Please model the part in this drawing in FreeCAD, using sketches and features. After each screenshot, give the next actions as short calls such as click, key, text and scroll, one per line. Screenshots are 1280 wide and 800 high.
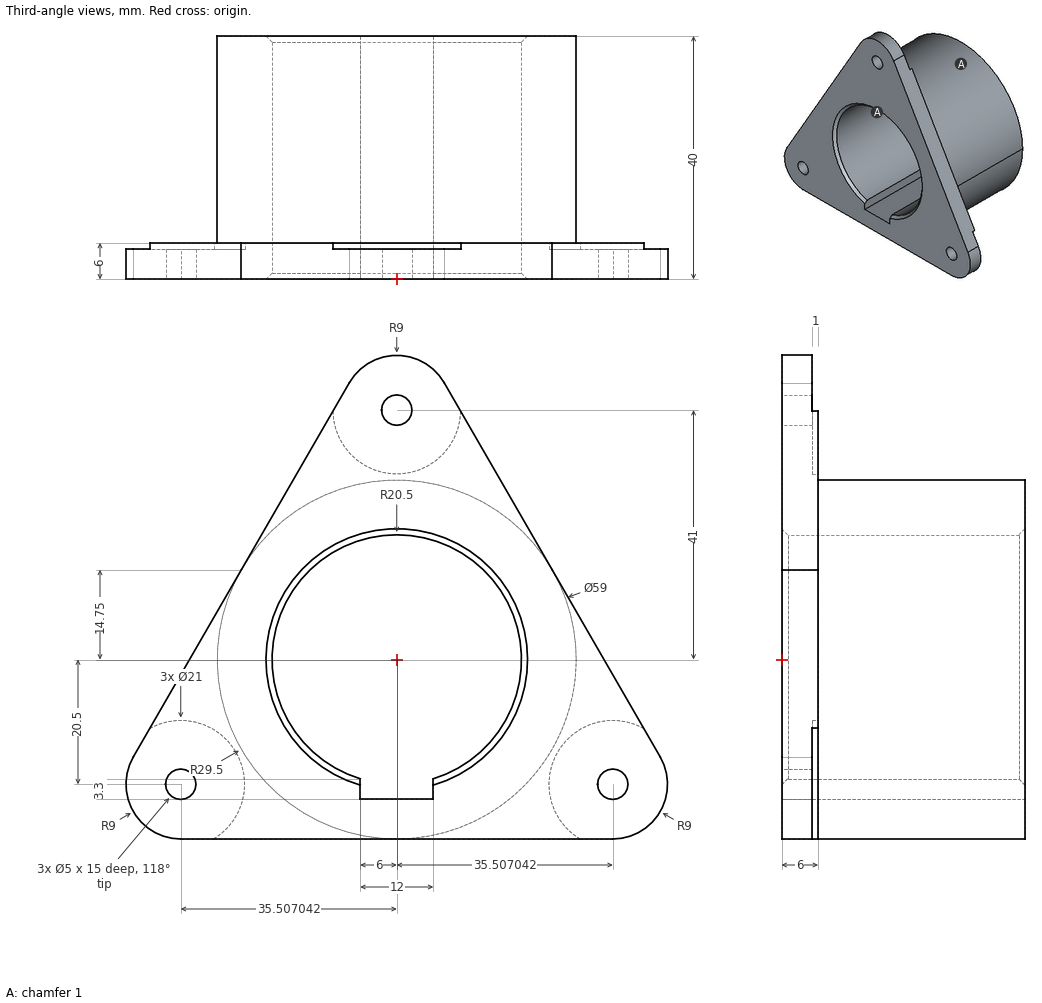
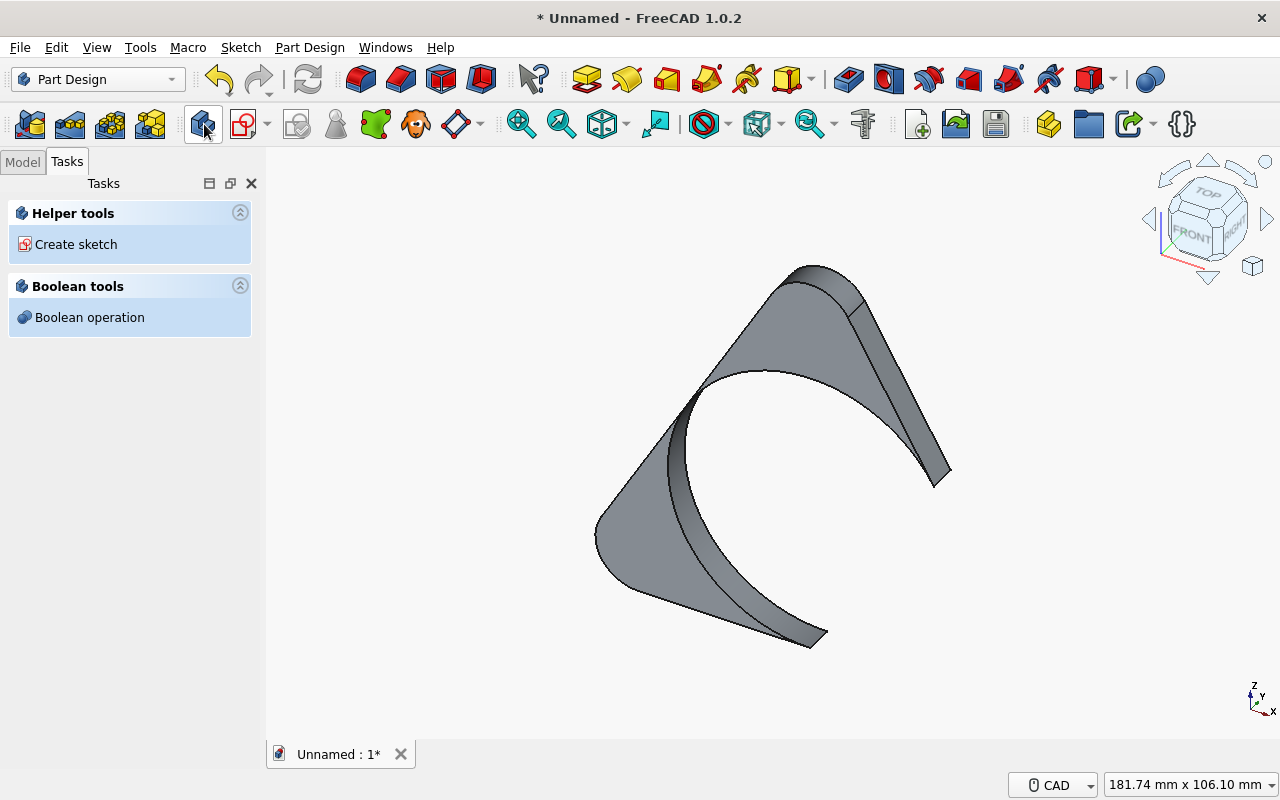
click(306, 699)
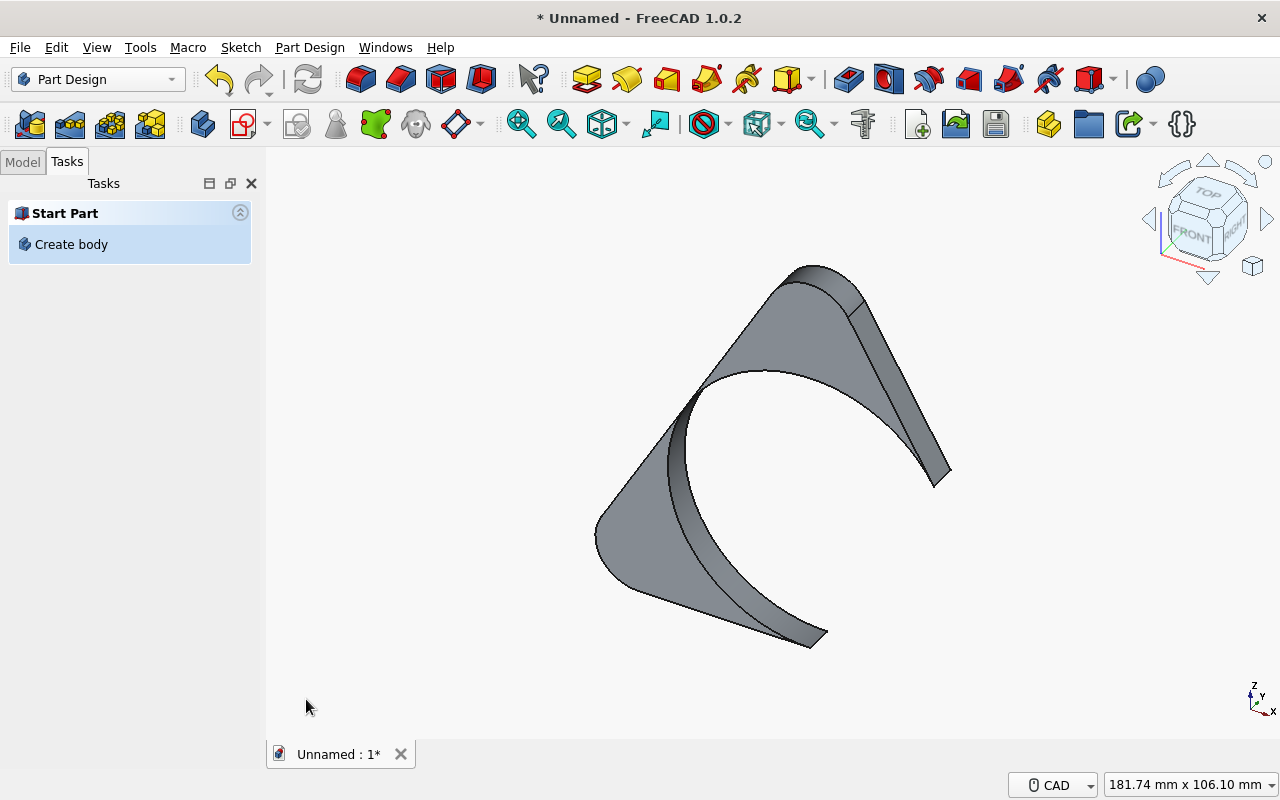
click(244, 124)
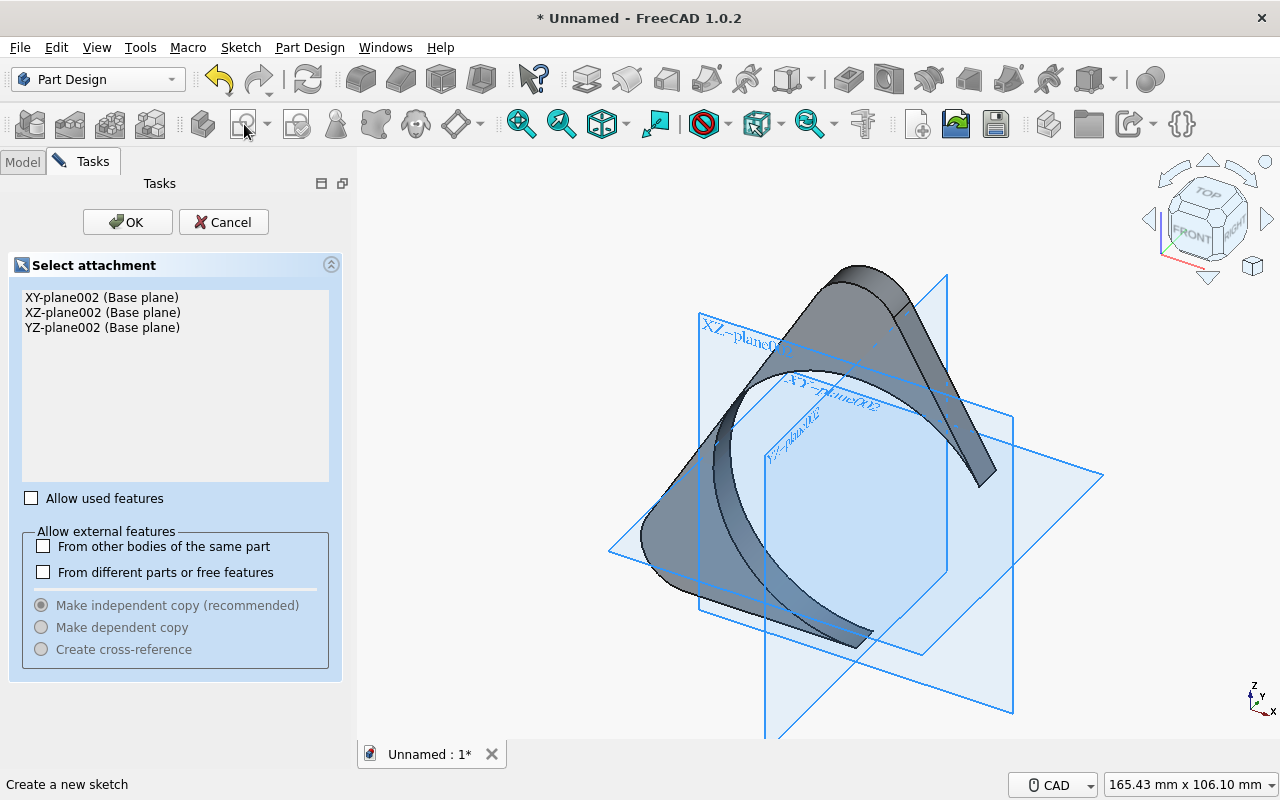
click(82, 312)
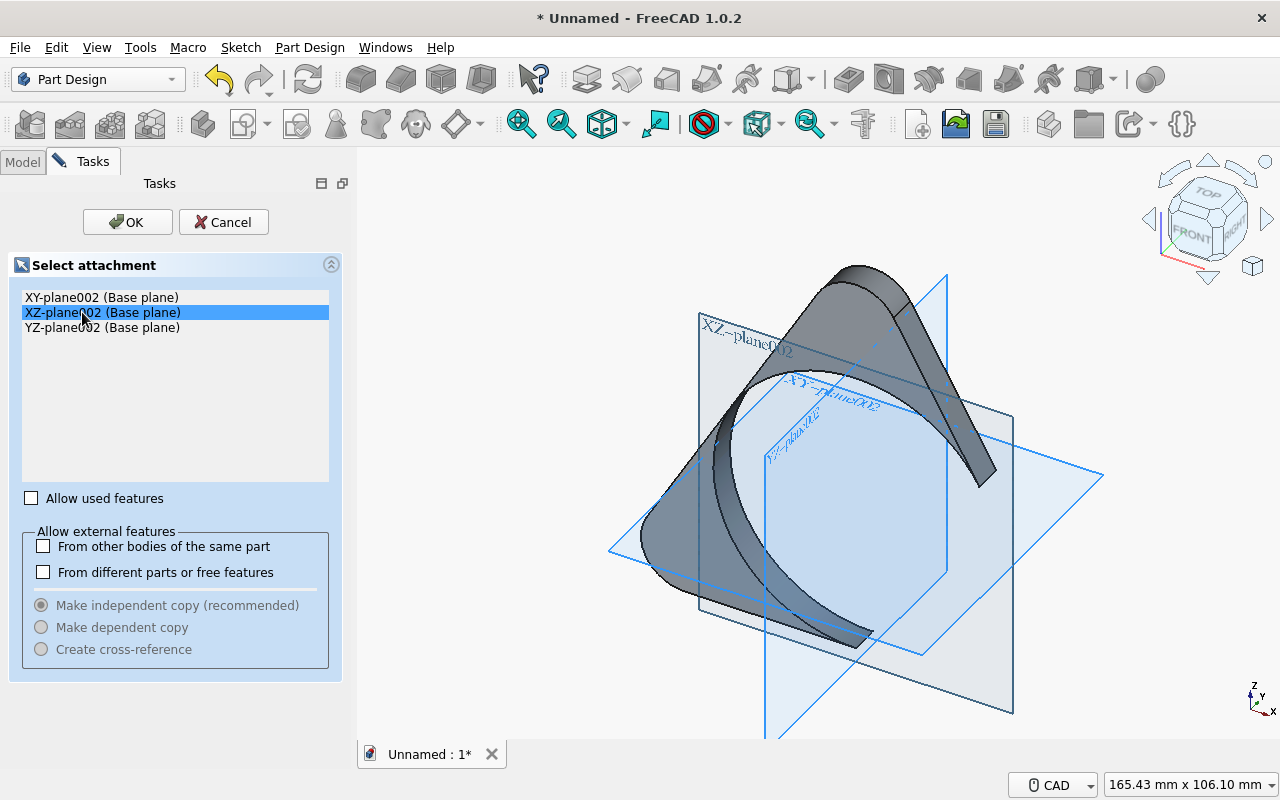
click(128, 222)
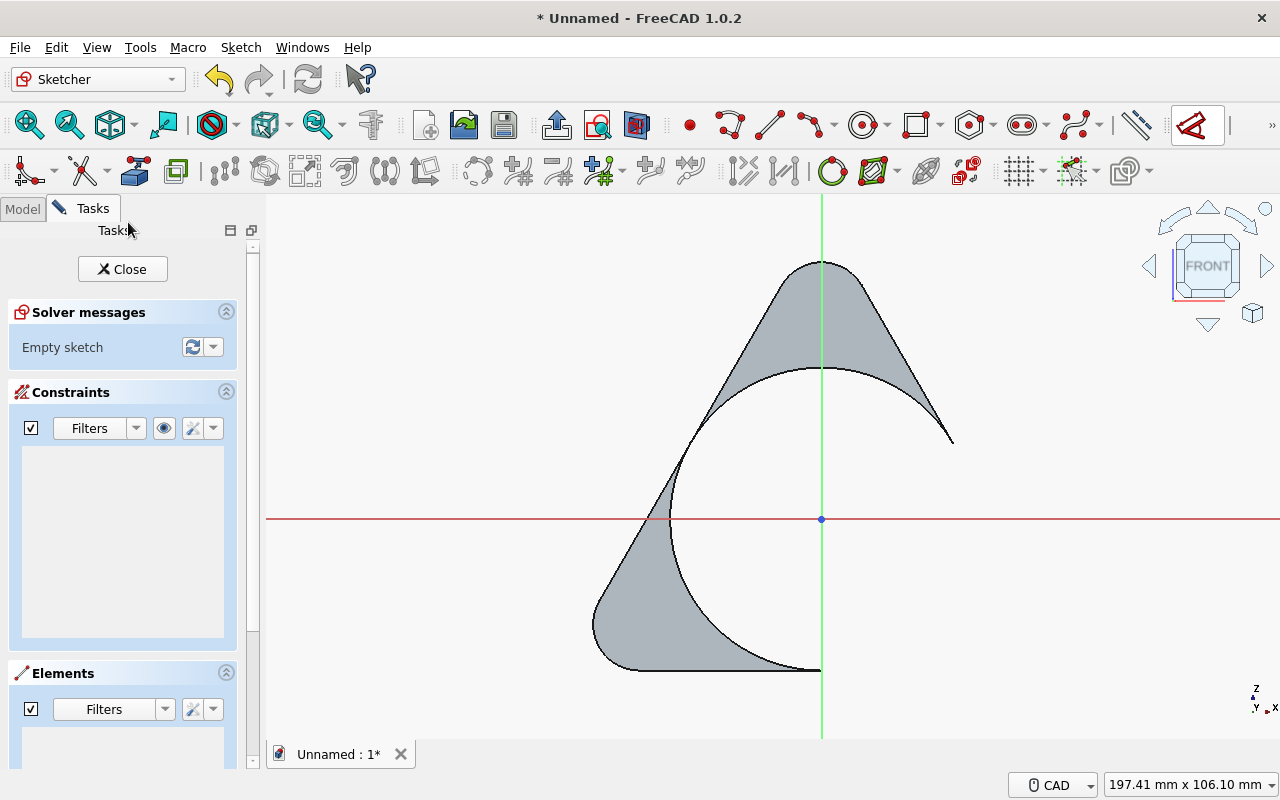
scroll(1115, 711, up, 2)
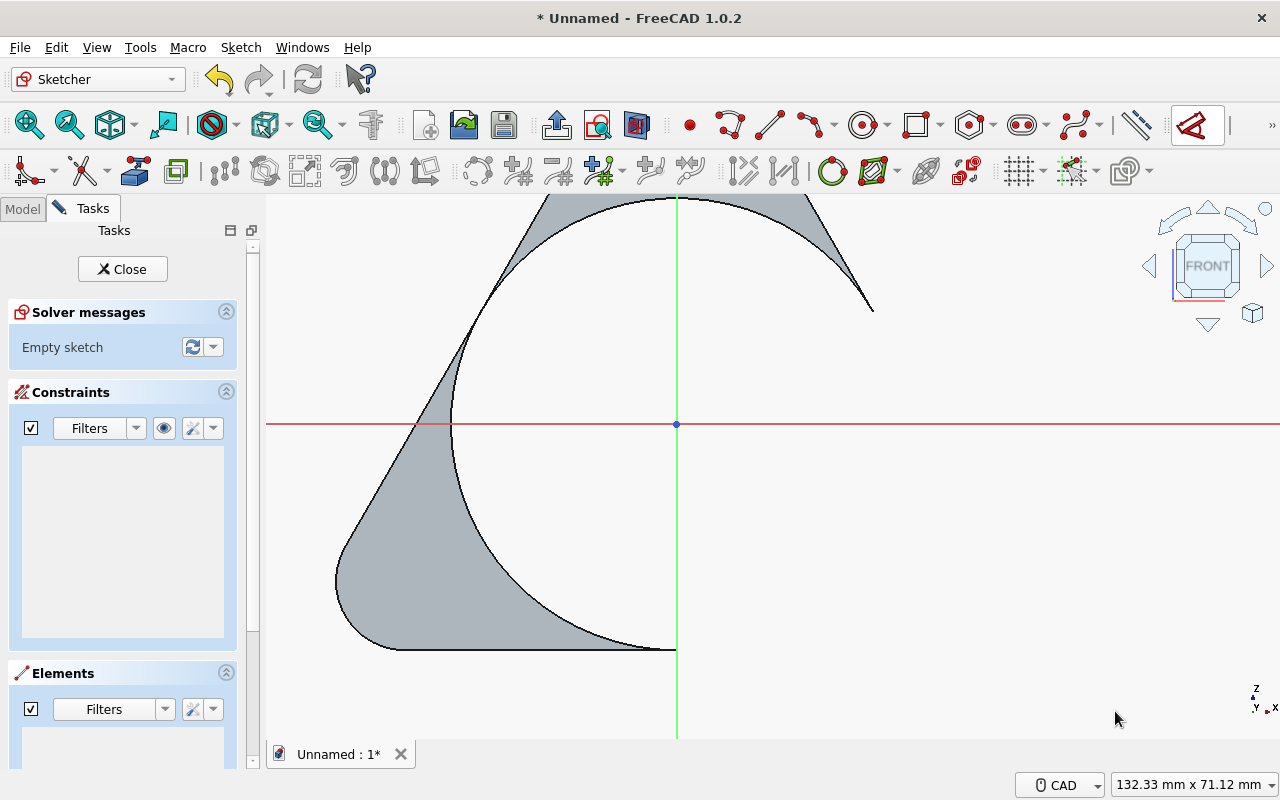
click(770, 126)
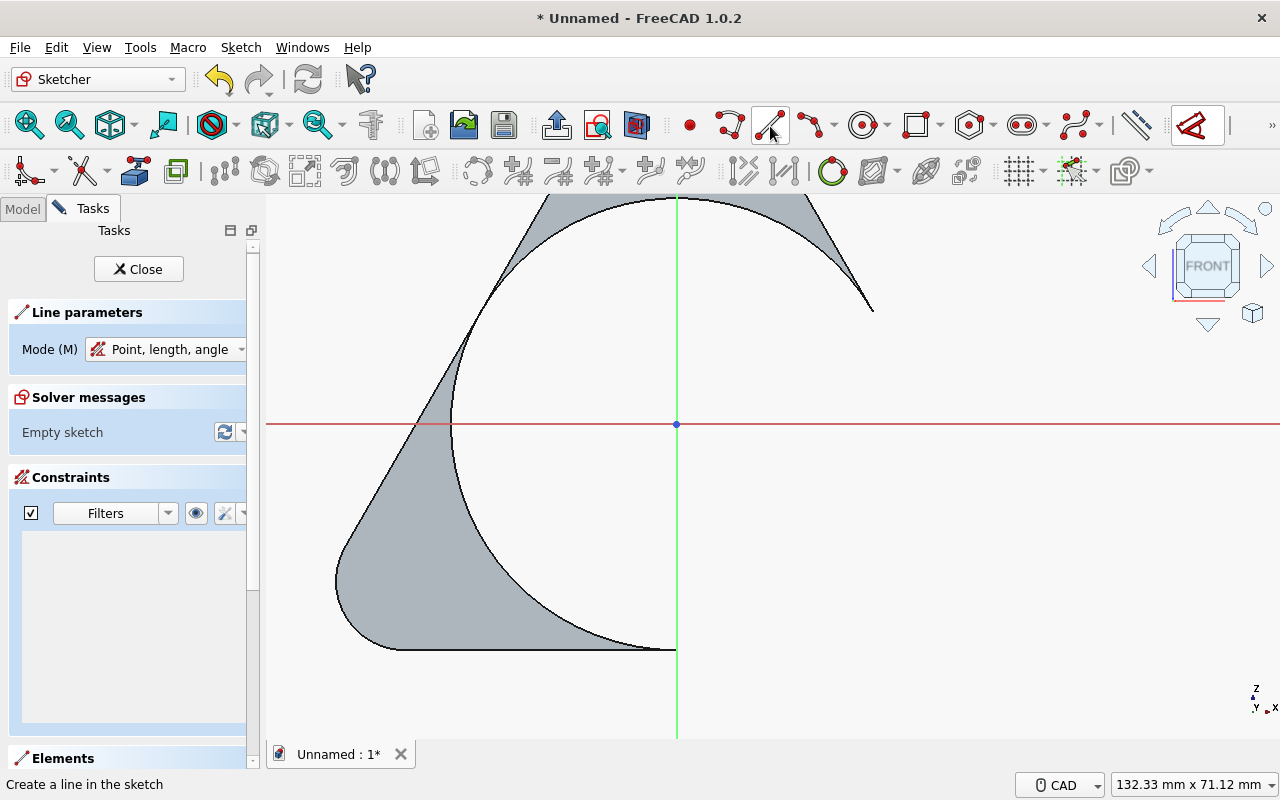
click(949, 650)
click(677, 650)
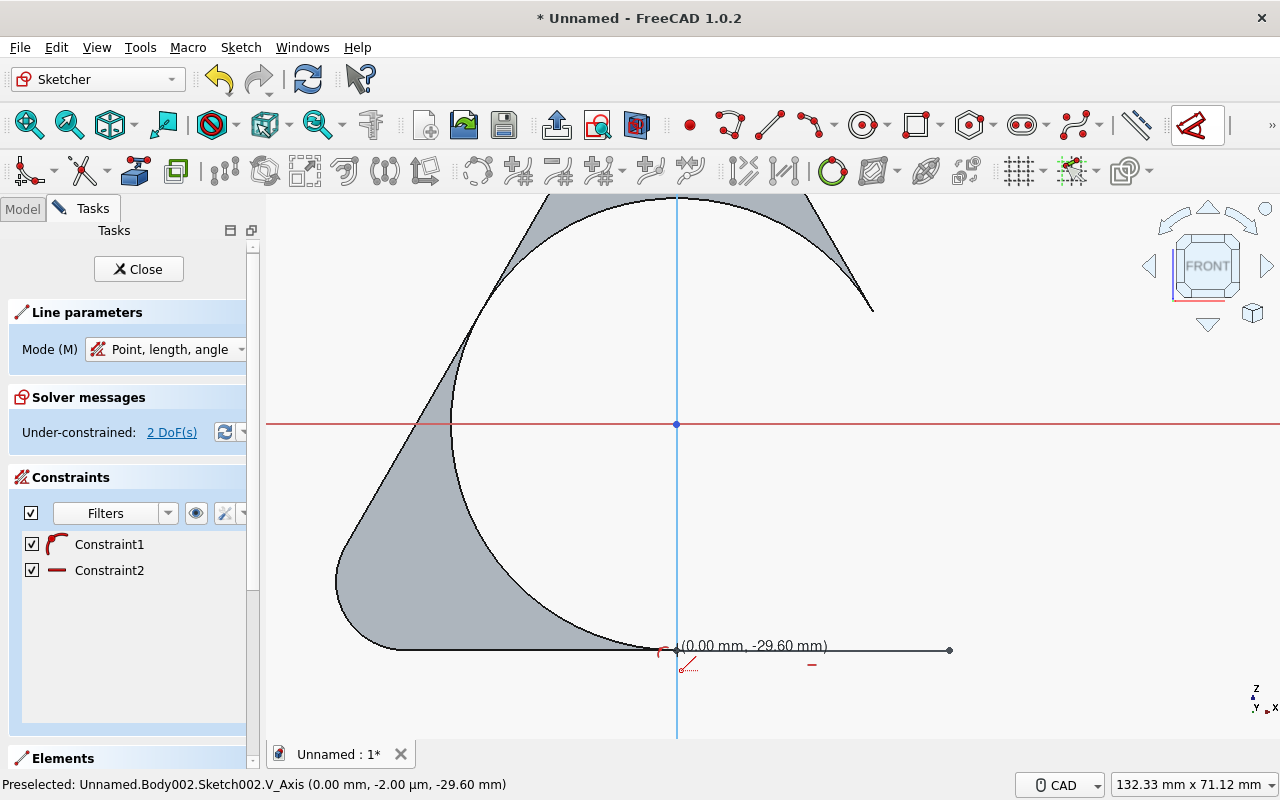
click(873, 311)
click(1009, 547)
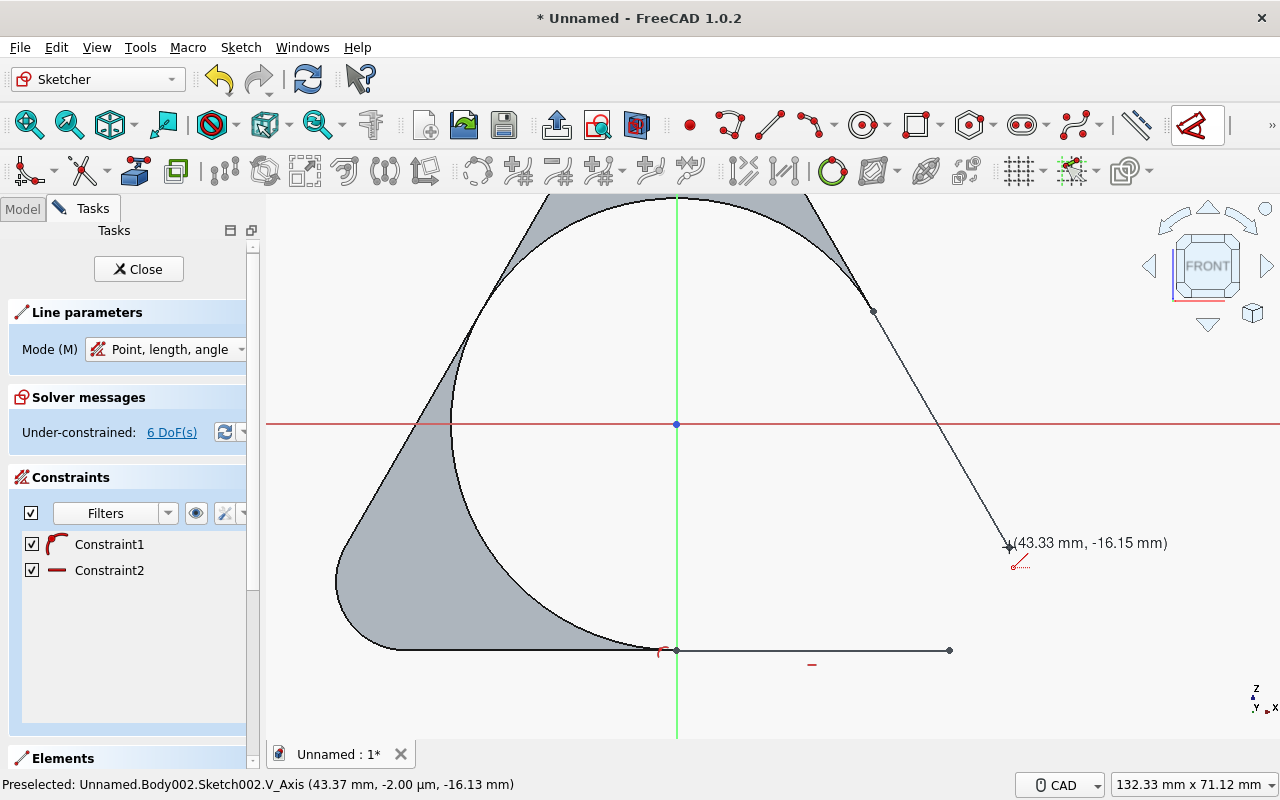
click(810, 126)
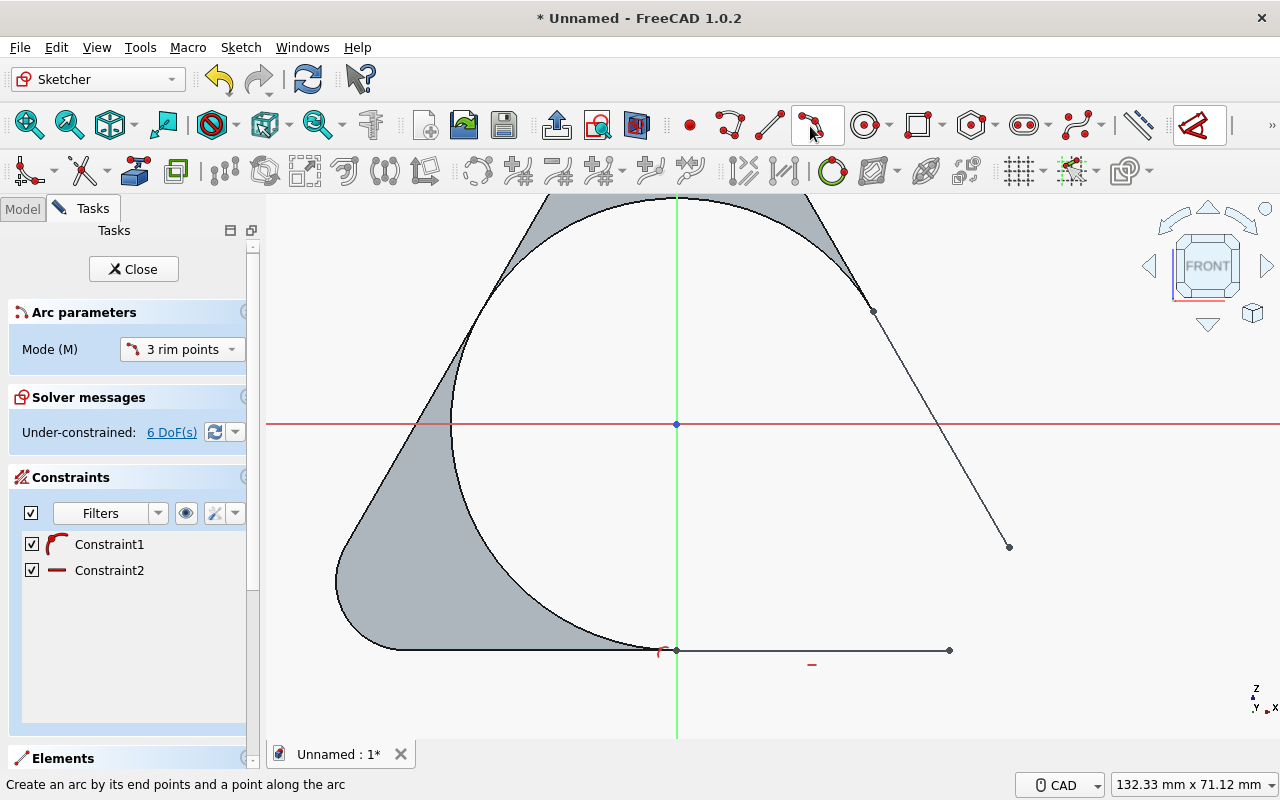
click(677, 651)
click(873, 312)
click(873, 537)